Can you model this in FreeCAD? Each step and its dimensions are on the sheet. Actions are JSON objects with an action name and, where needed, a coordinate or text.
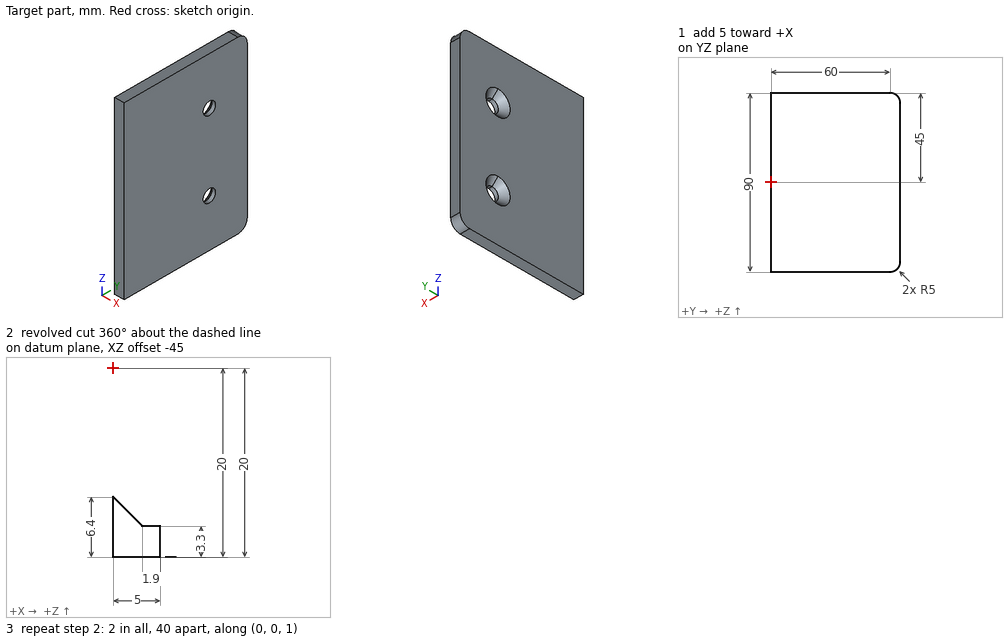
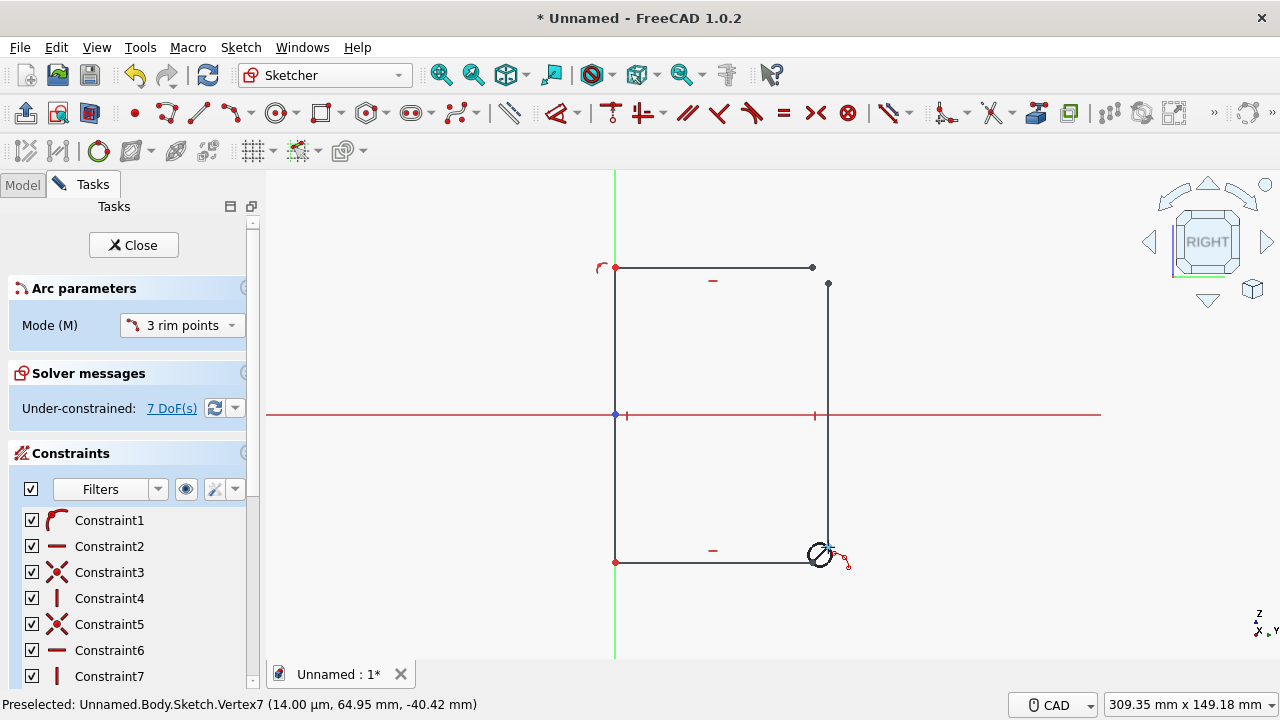
{"action": "scroll", "coordinate": [823, 557], "scroll_direction": "up", "scroll_amount": 6}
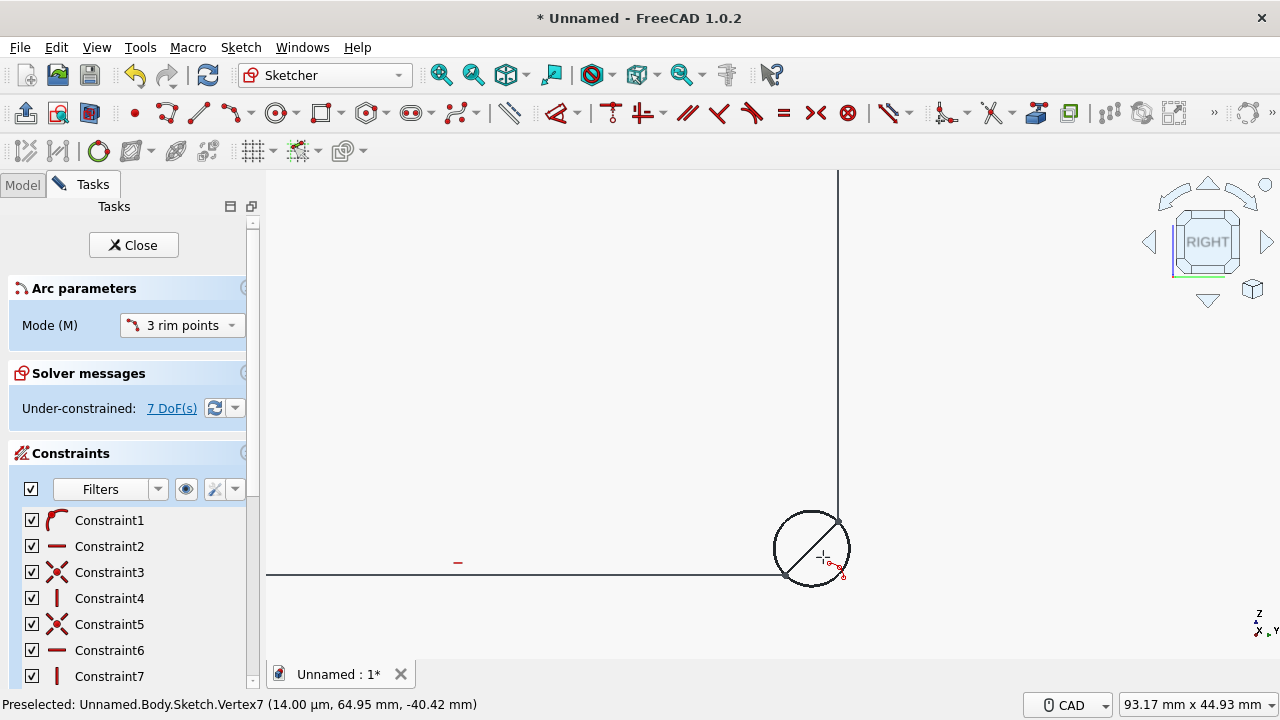
{"action": "left_click", "coordinate": [823, 556]}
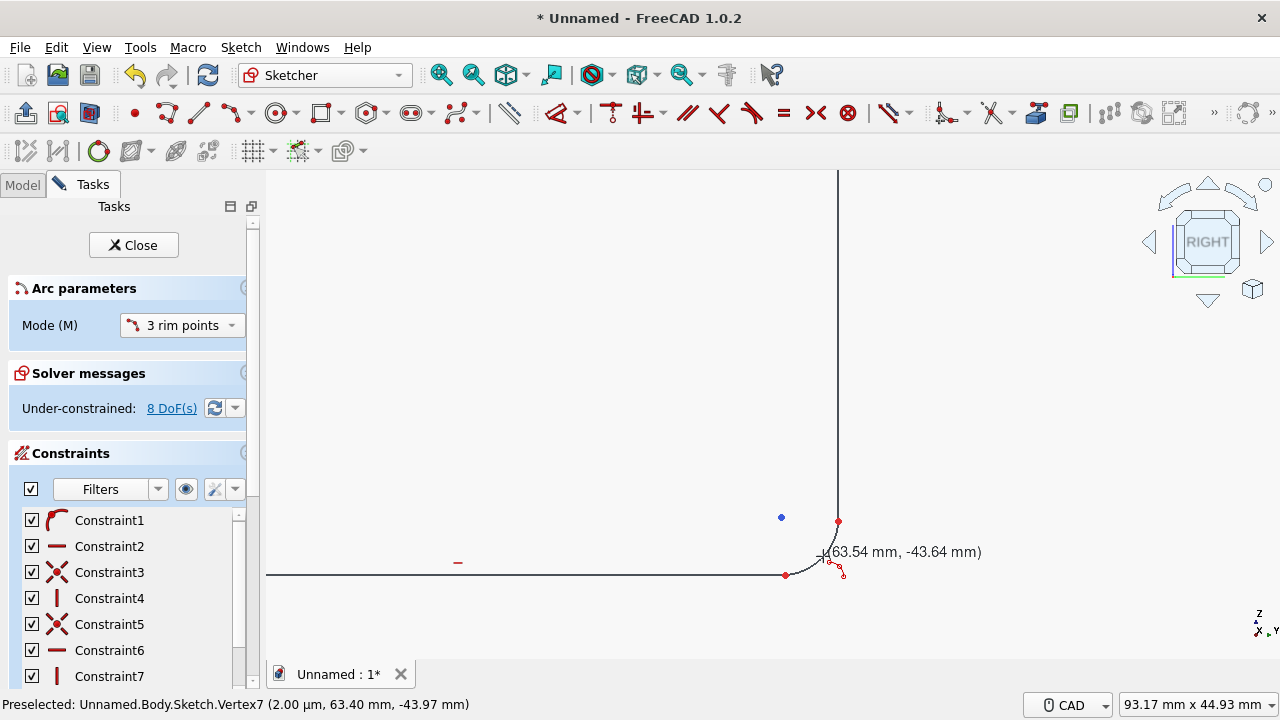
{"action": "scroll", "coordinate": [799, 558], "scroll_direction": "down", "scroll_amount": 6}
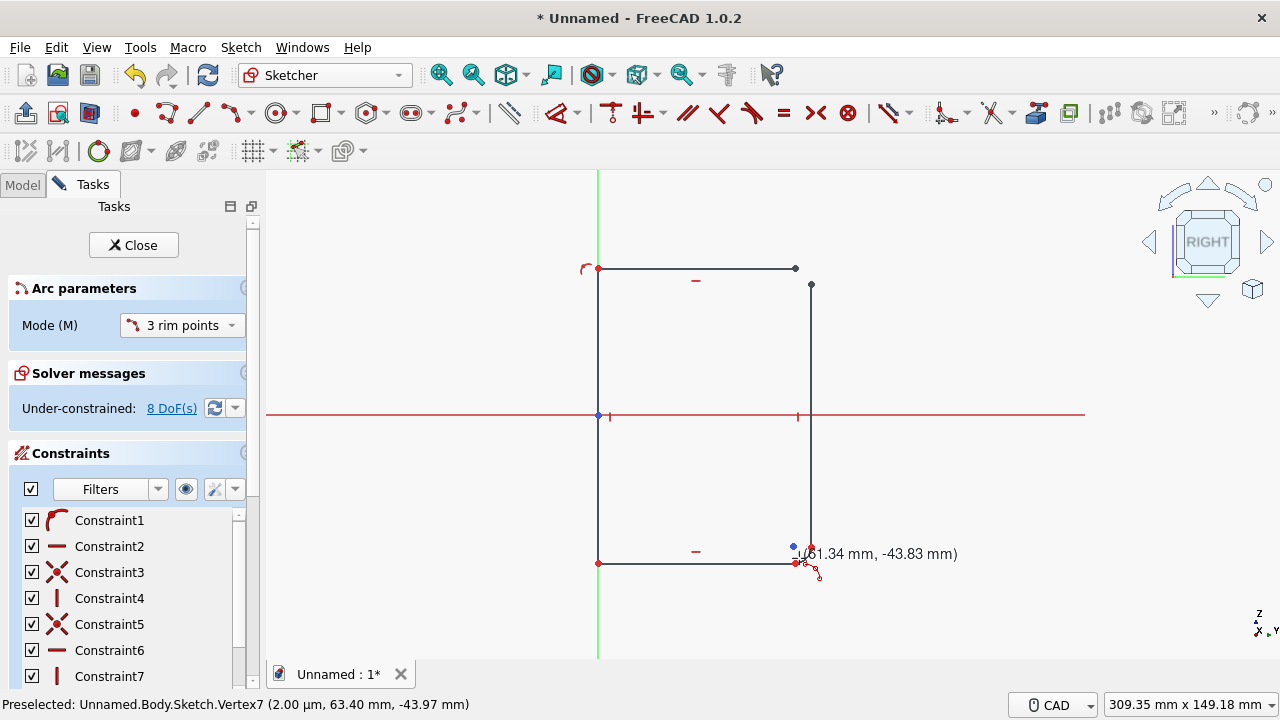
{"action": "left_click", "coordinate": [811, 285]}
{"action": "left_click", "coordinate": [795, 269]}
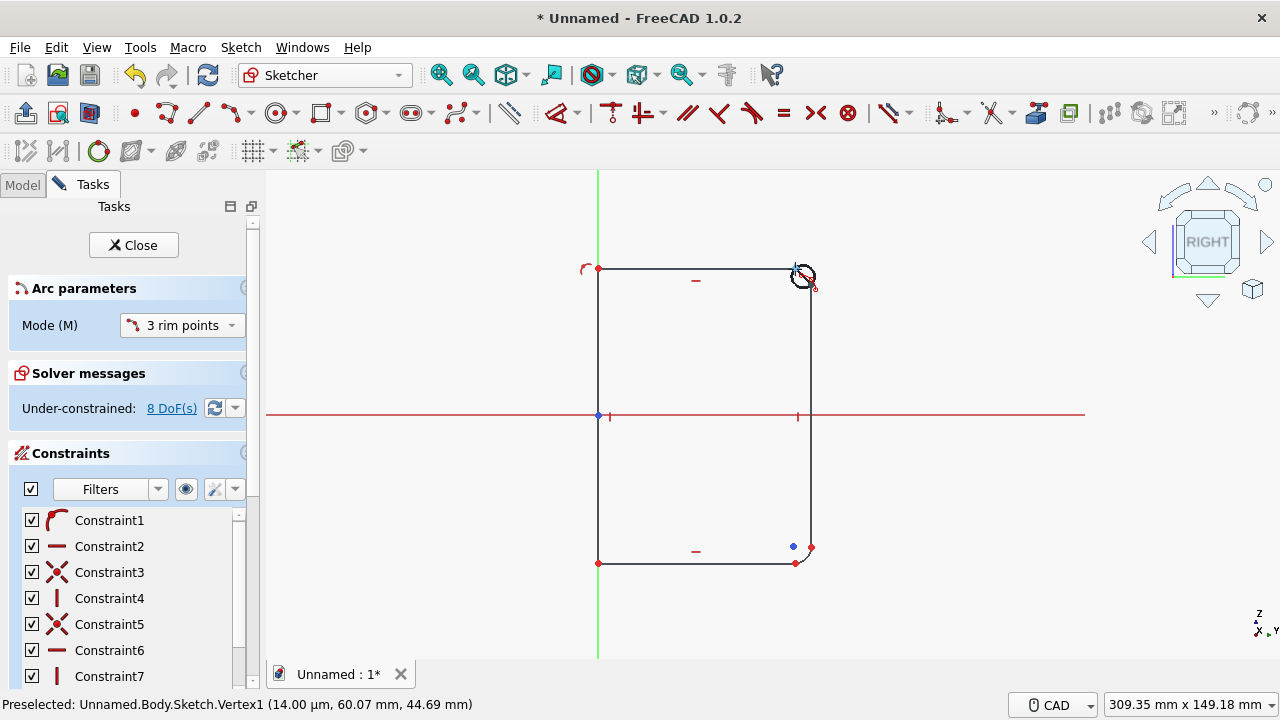
{"action": "scroll", "coordinate": [807, 272], "scroll_direction": "up", "scroll_amount": 6}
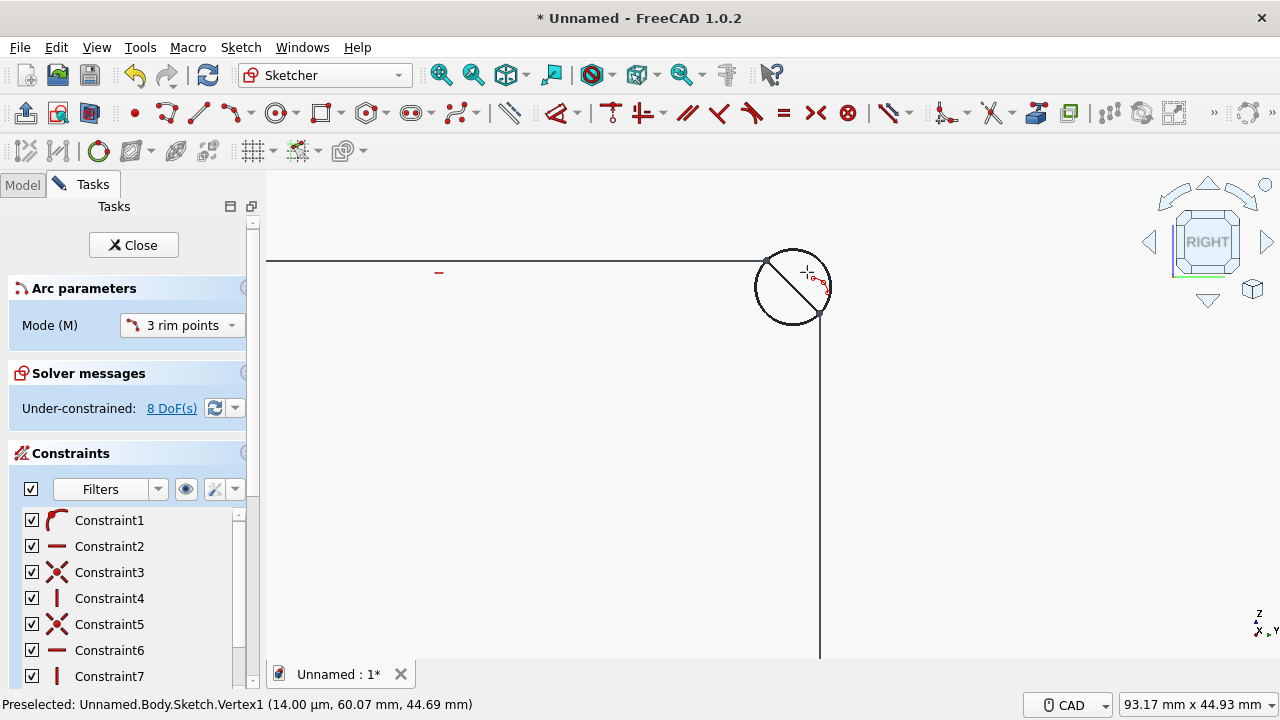
{"action": "left_click", "coordinate": [804, 273]}
{"action": "key", "text": "Escape"}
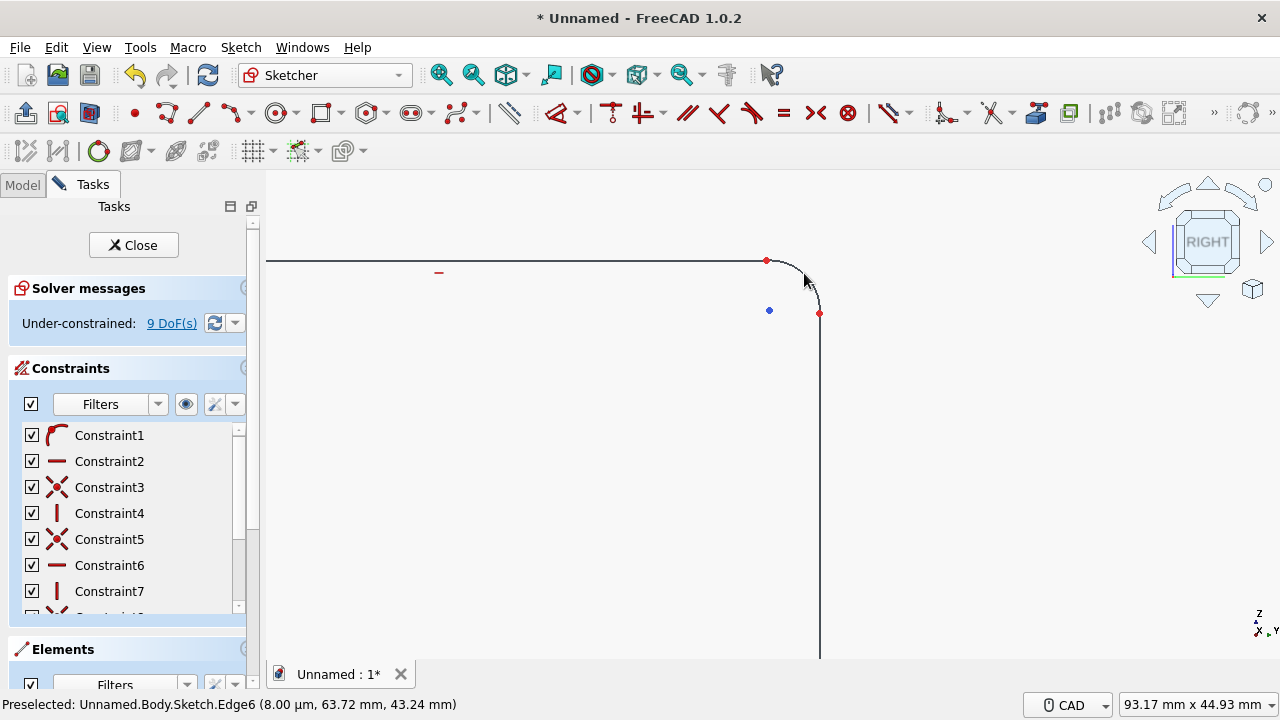
{"action": "left_click", "coordinate": [570, 261]}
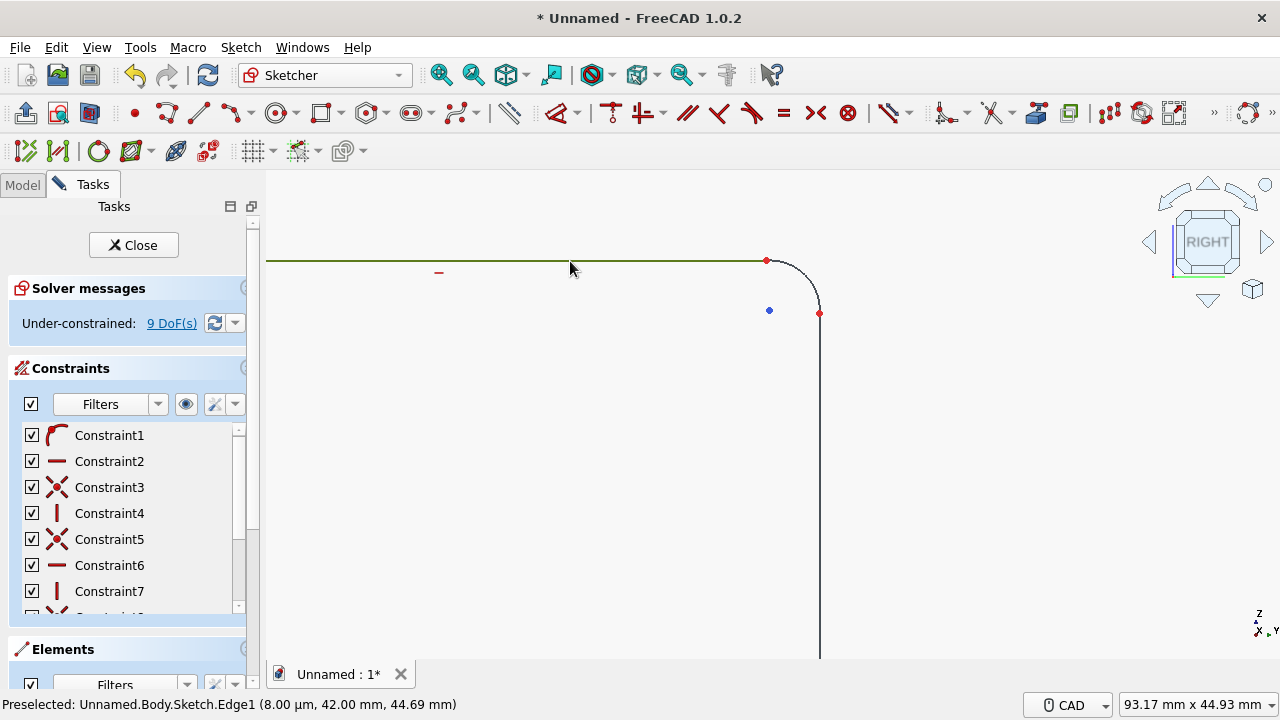
{"action": "left_click", "coordinate": [815, 289]}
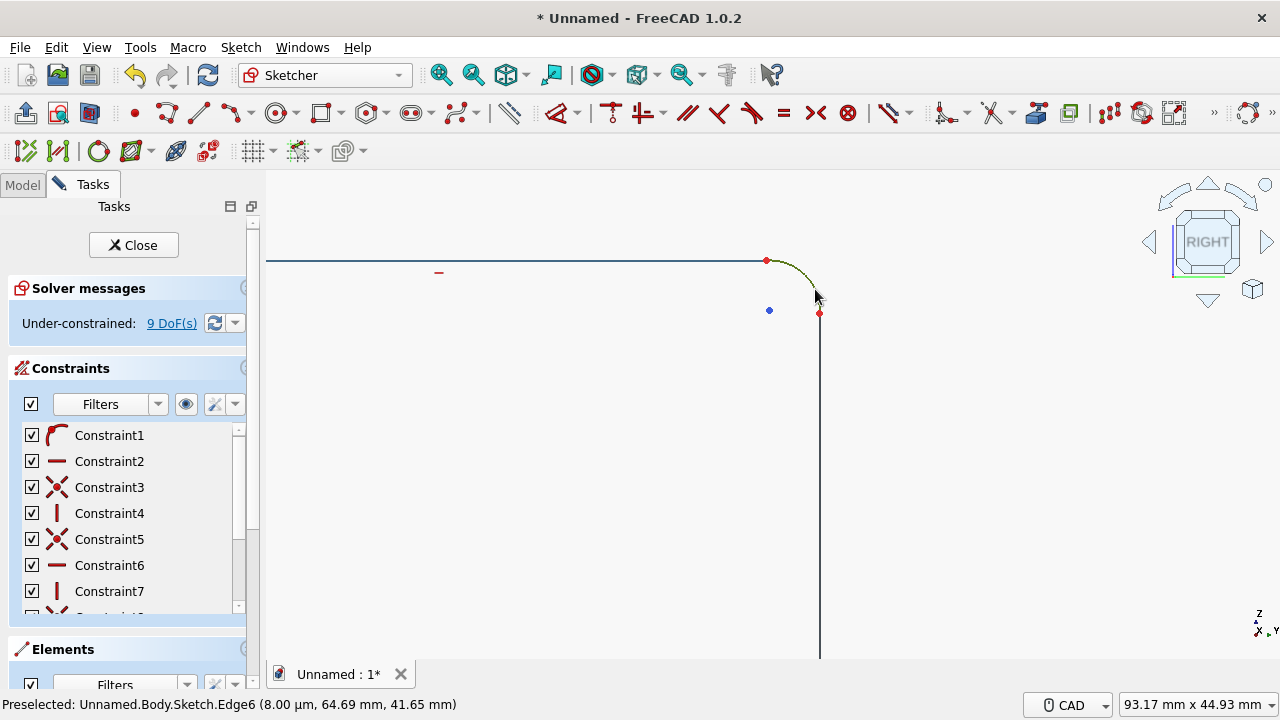
{"action": "left_click", "coordinate": [752, 114]}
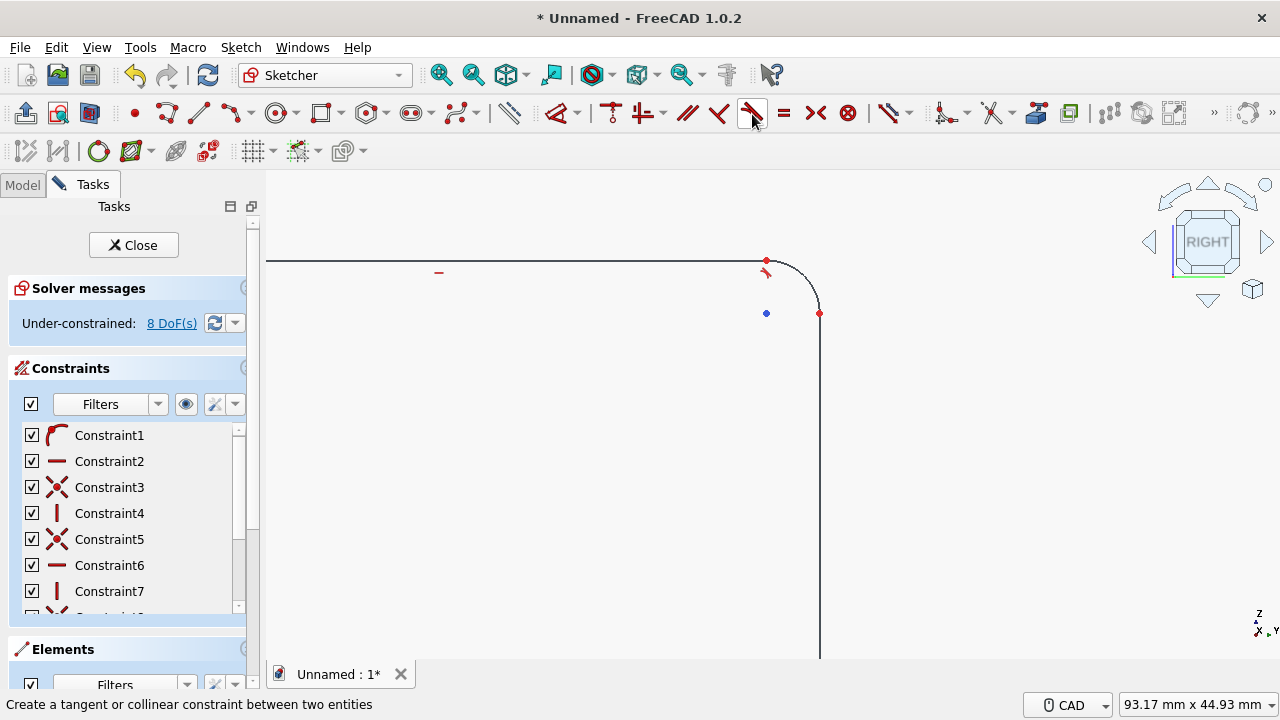
{"action": "scroll", "coordinate": [807, 271], "scroll_direction": "down", "scroll_amount": 6}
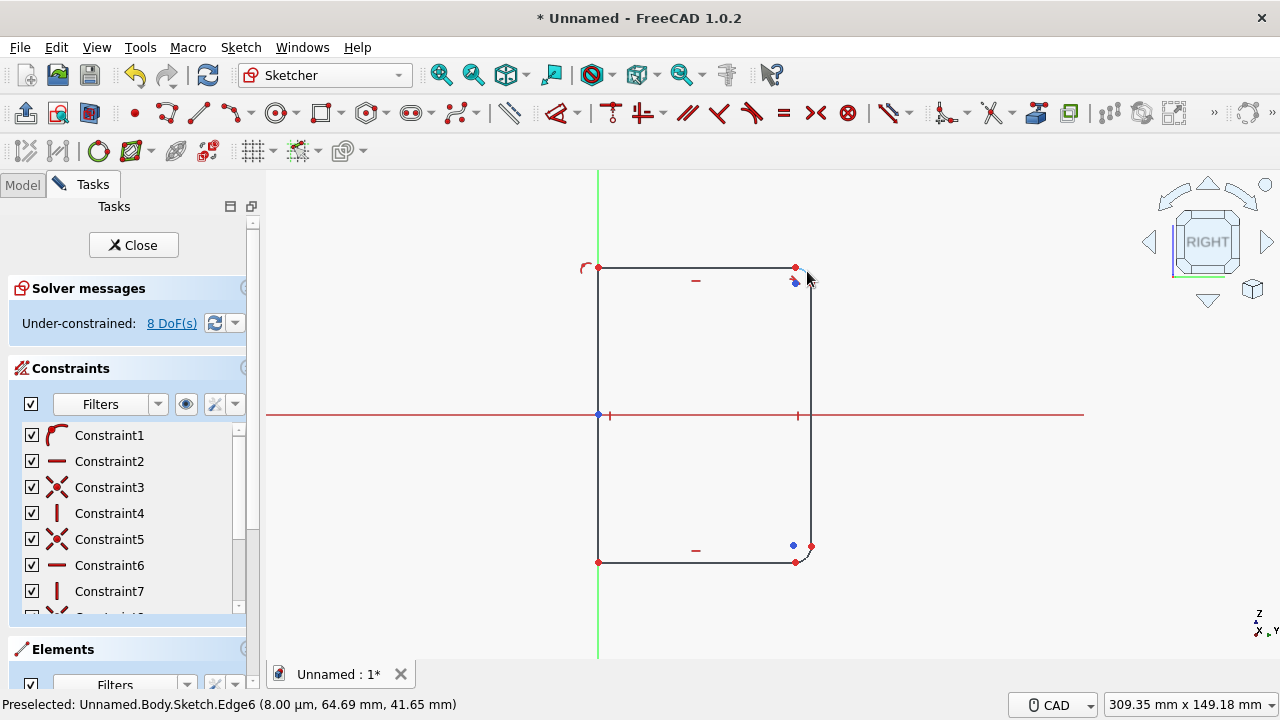
{"action": "left_click", "coordinate": [657, 563]}